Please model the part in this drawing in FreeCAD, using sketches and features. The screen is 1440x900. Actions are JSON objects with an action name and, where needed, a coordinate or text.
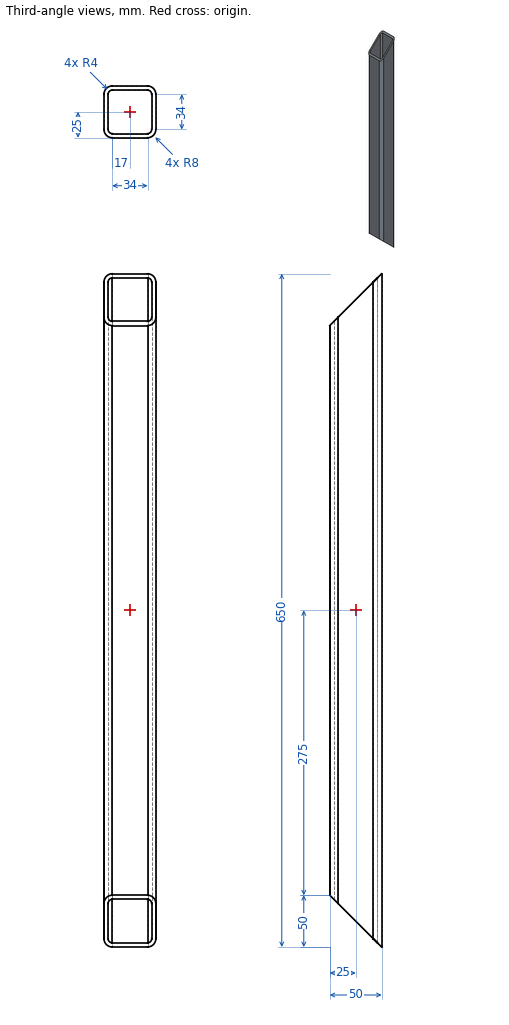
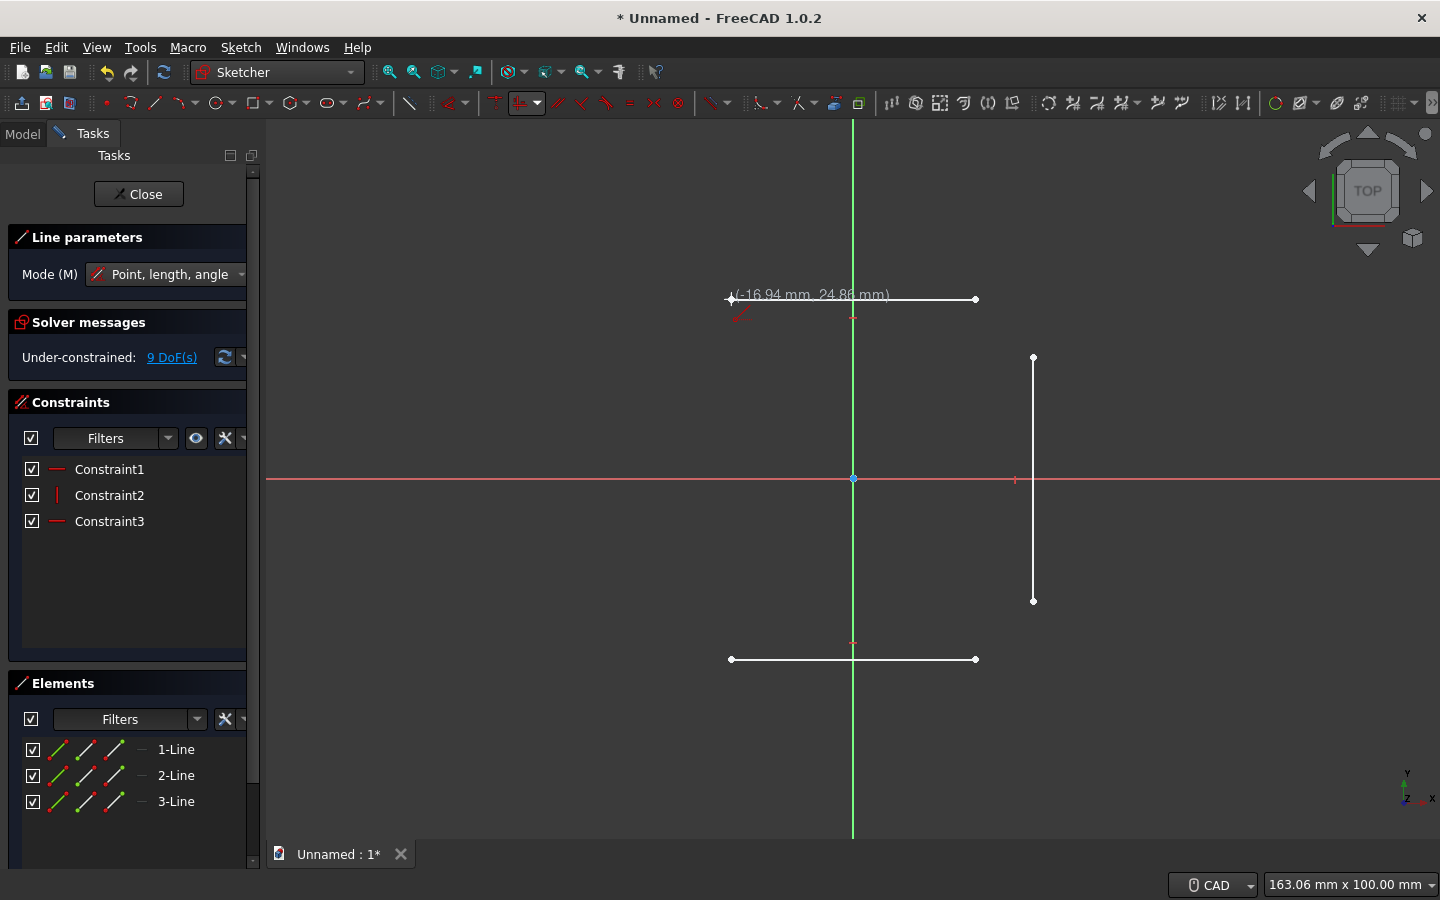
{"action": "left_click", "coordinate": [673, 357]}
{"action": "left_click", "coordinate": [673, 601]}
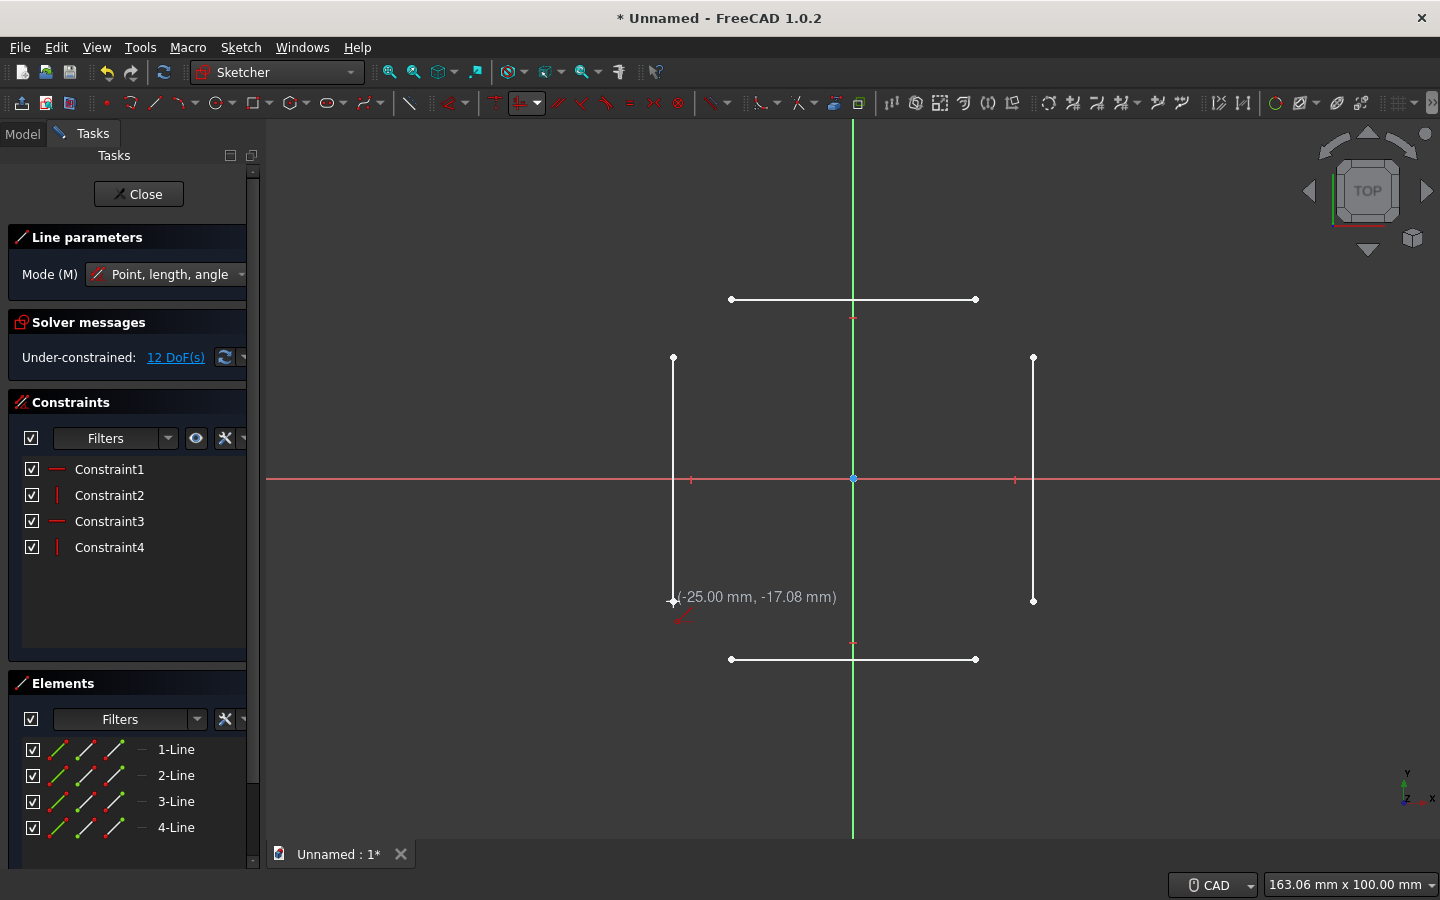
{"action": "key", "text": "g 3 a"}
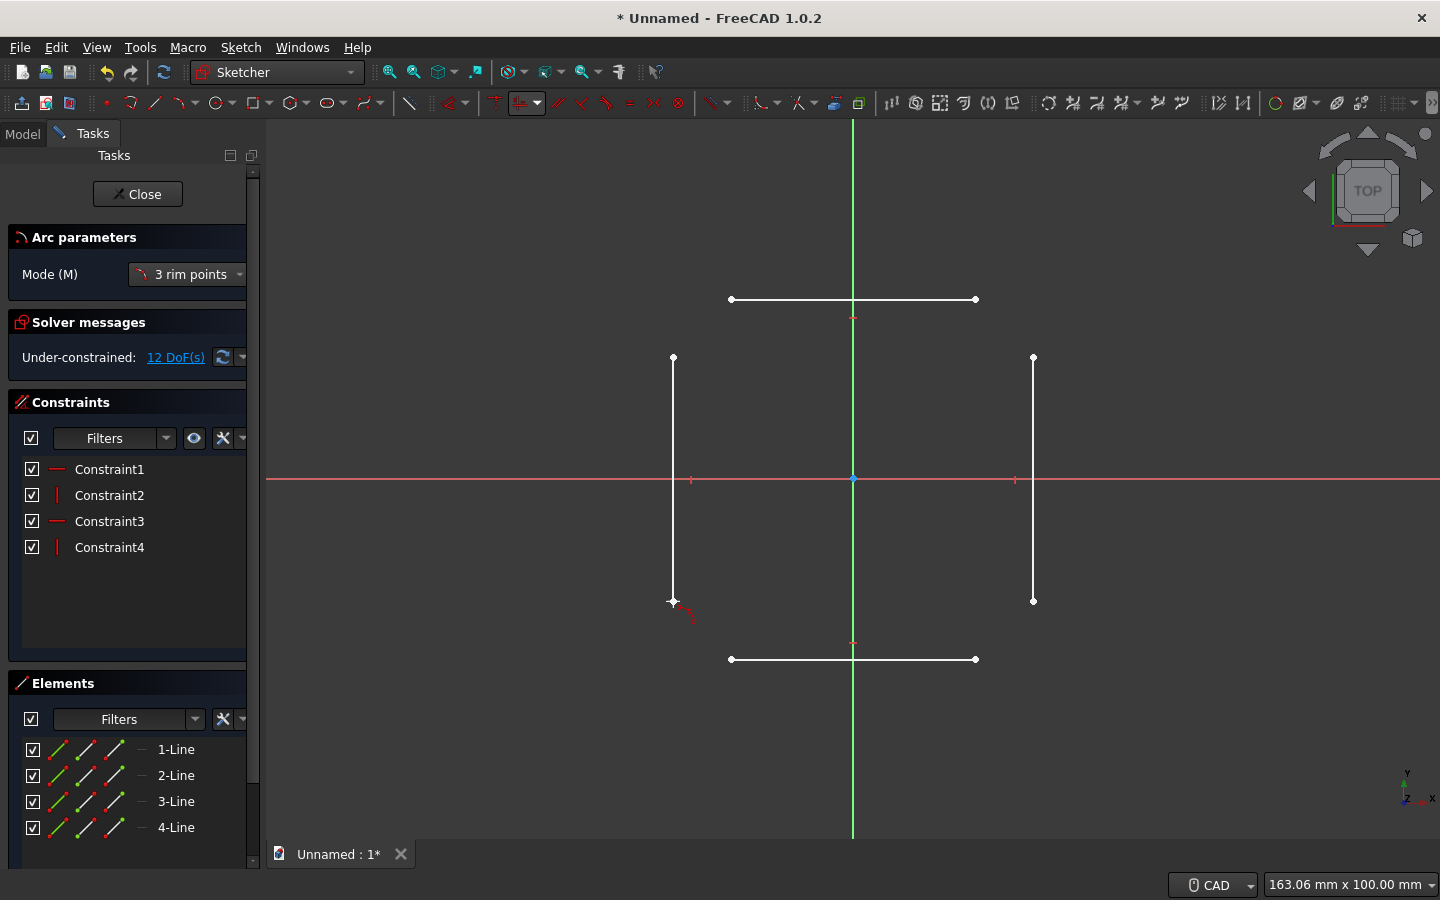
{"action": "left_click", "coordinate": [975, 660]}
{"action": "left_click", "coordinate": [1033, 602]}
{"action": "left_click", "coordinate": [1016, 642]}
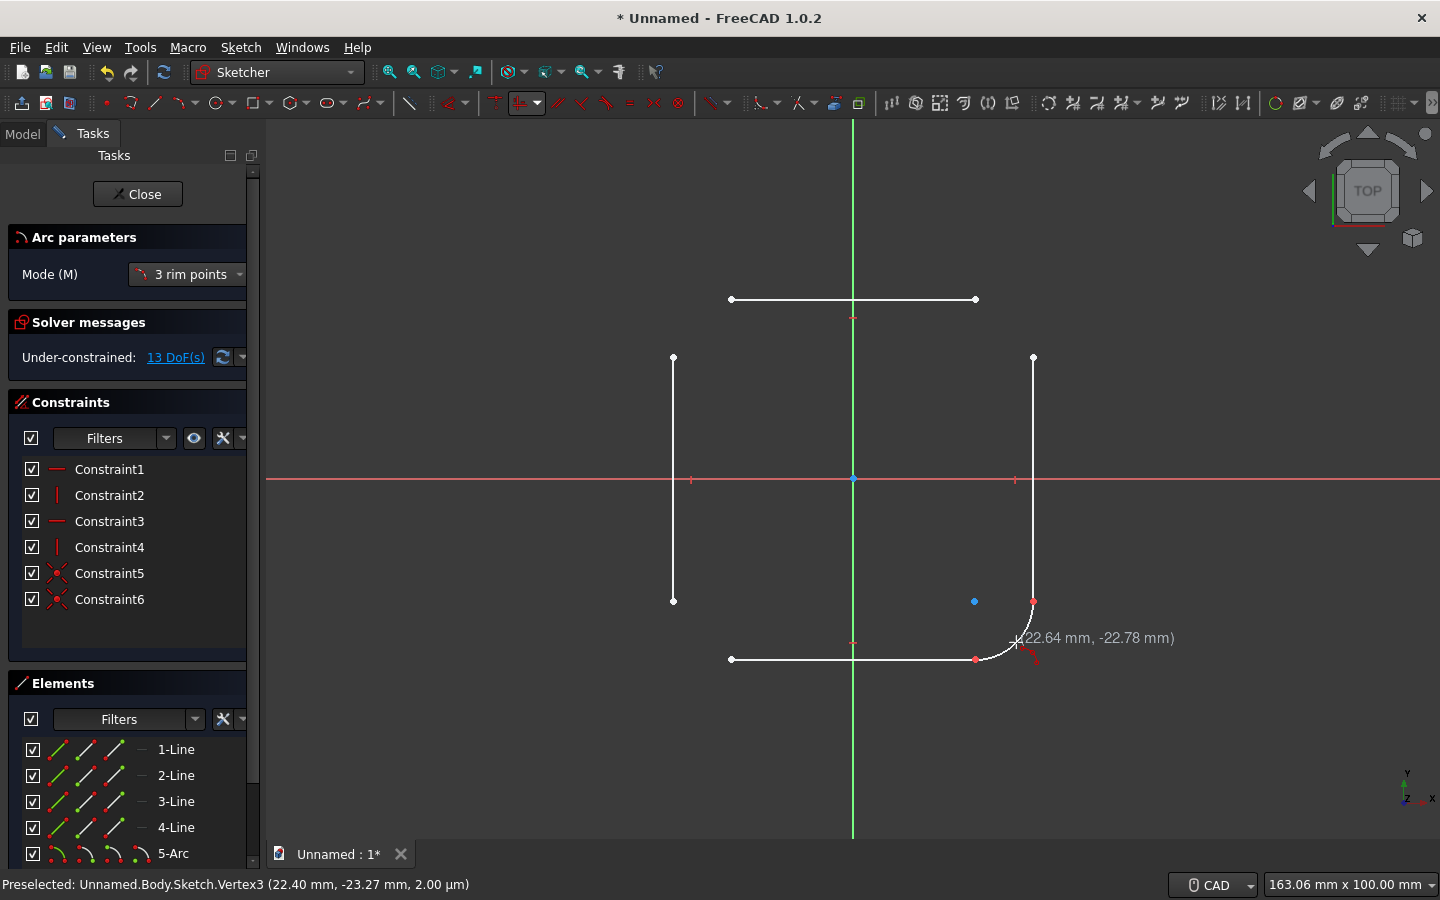
{"action": "left_click", "coordinate": [1033, 358]}
{"action": "left_click", "coordinate": [975, 300]}
{"action": "left_click", "coordinate": [1016, 316]}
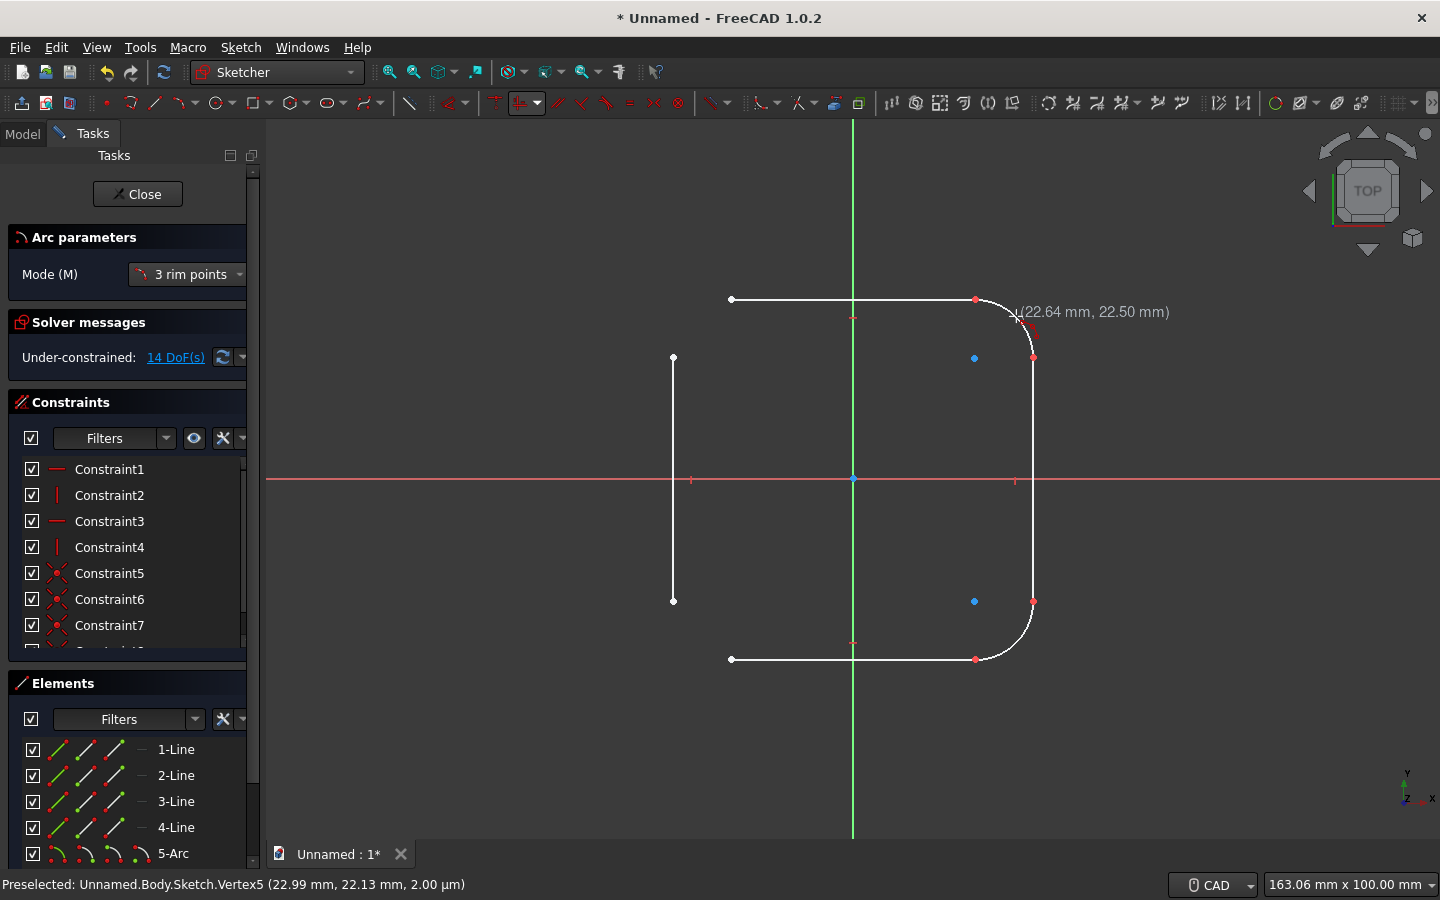
{"action": "left_click", "coordinate": [731, 300]}
{"action": "left_click", "coordinate": [673, 358]}
{"action": "left_click", "coordinate": [690, 316]}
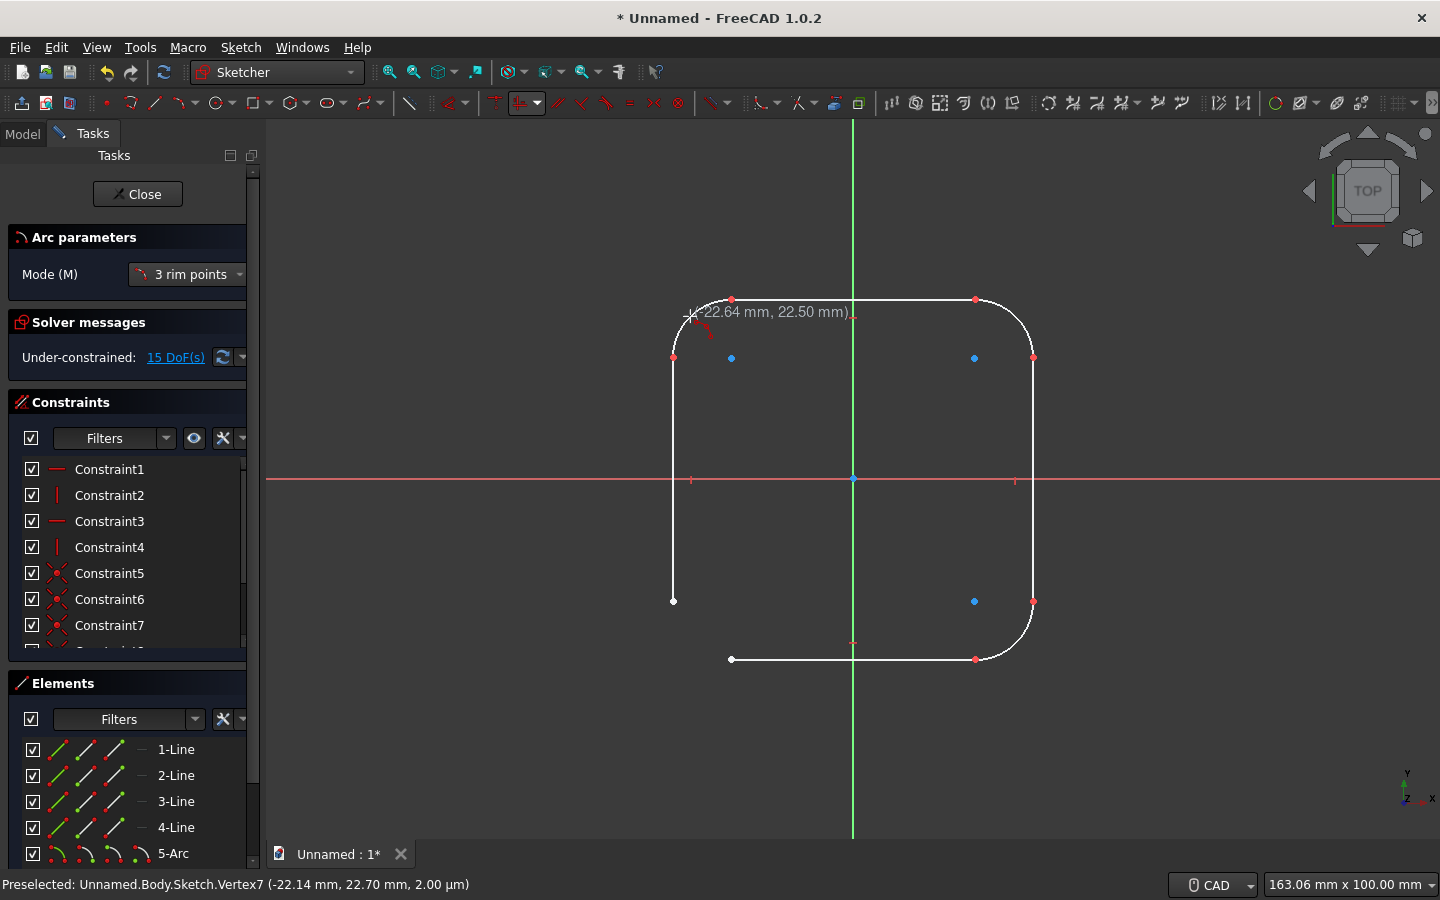
{"action": "left_click", "coordinate": [673, 602]}
{"action": "left_click", "coordinate": [731, 660]}
{"action": "left_click", "coordinate": [690, 642]}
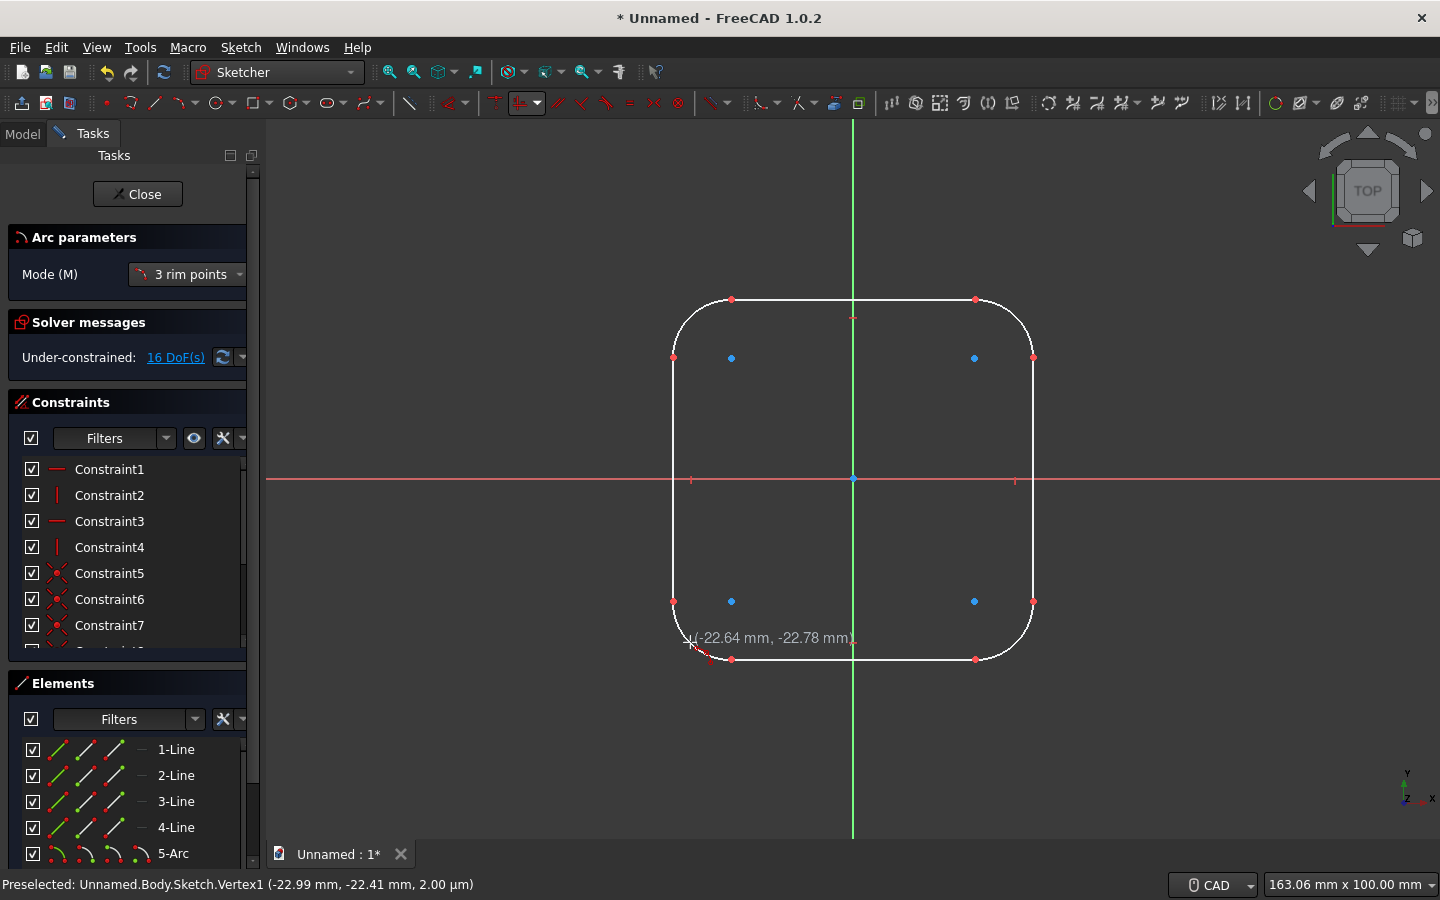
{"action": "left_click", "coordinate": [156, 104]}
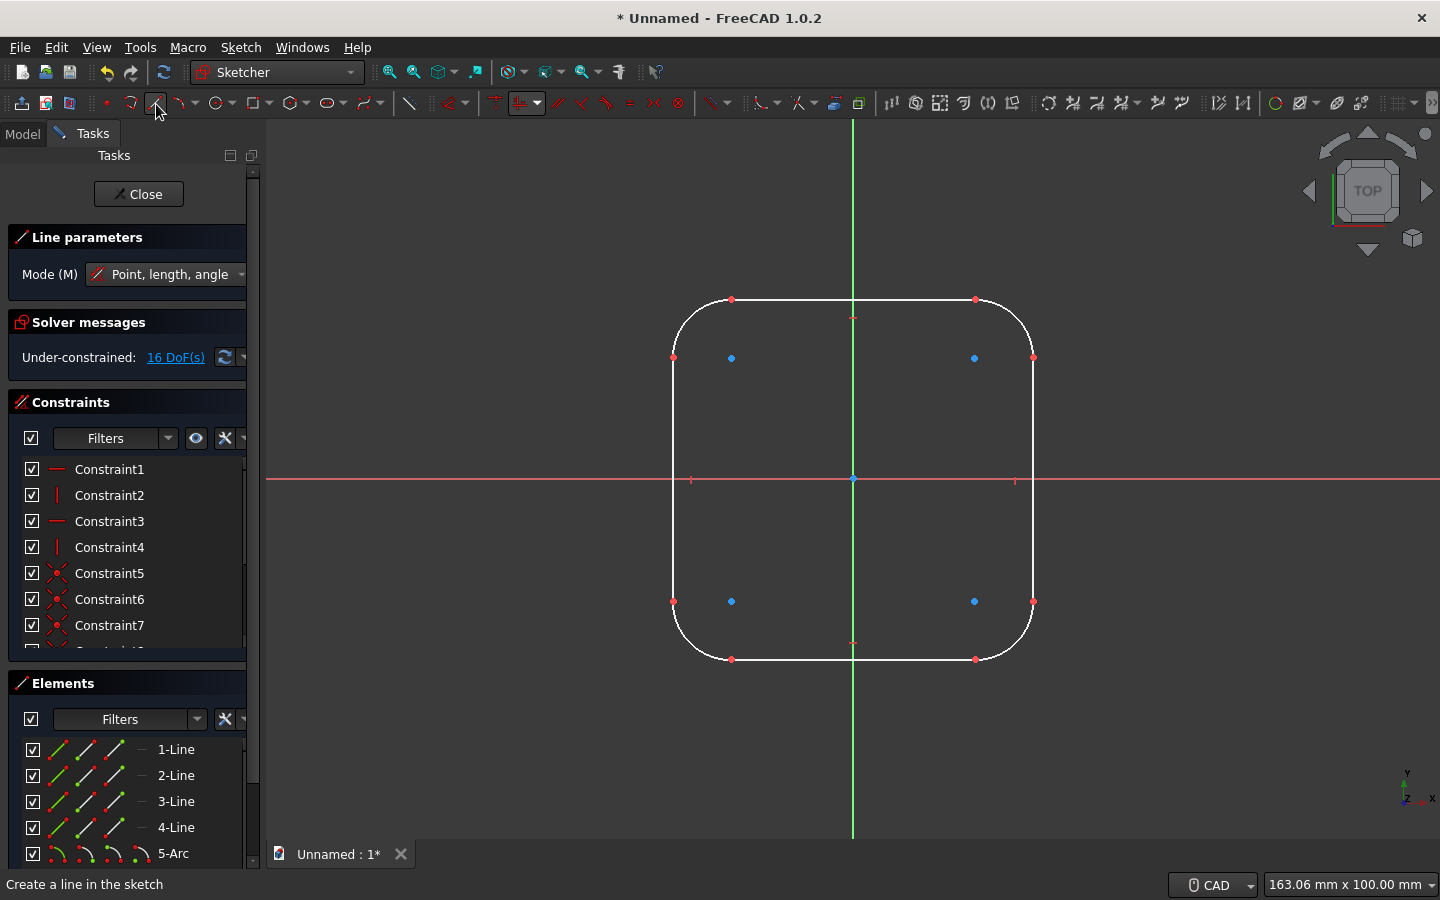
{"action": "left_click", "coordinate": [731, 328]}
{"action": "left_click", "coordinate": [975, 328]}